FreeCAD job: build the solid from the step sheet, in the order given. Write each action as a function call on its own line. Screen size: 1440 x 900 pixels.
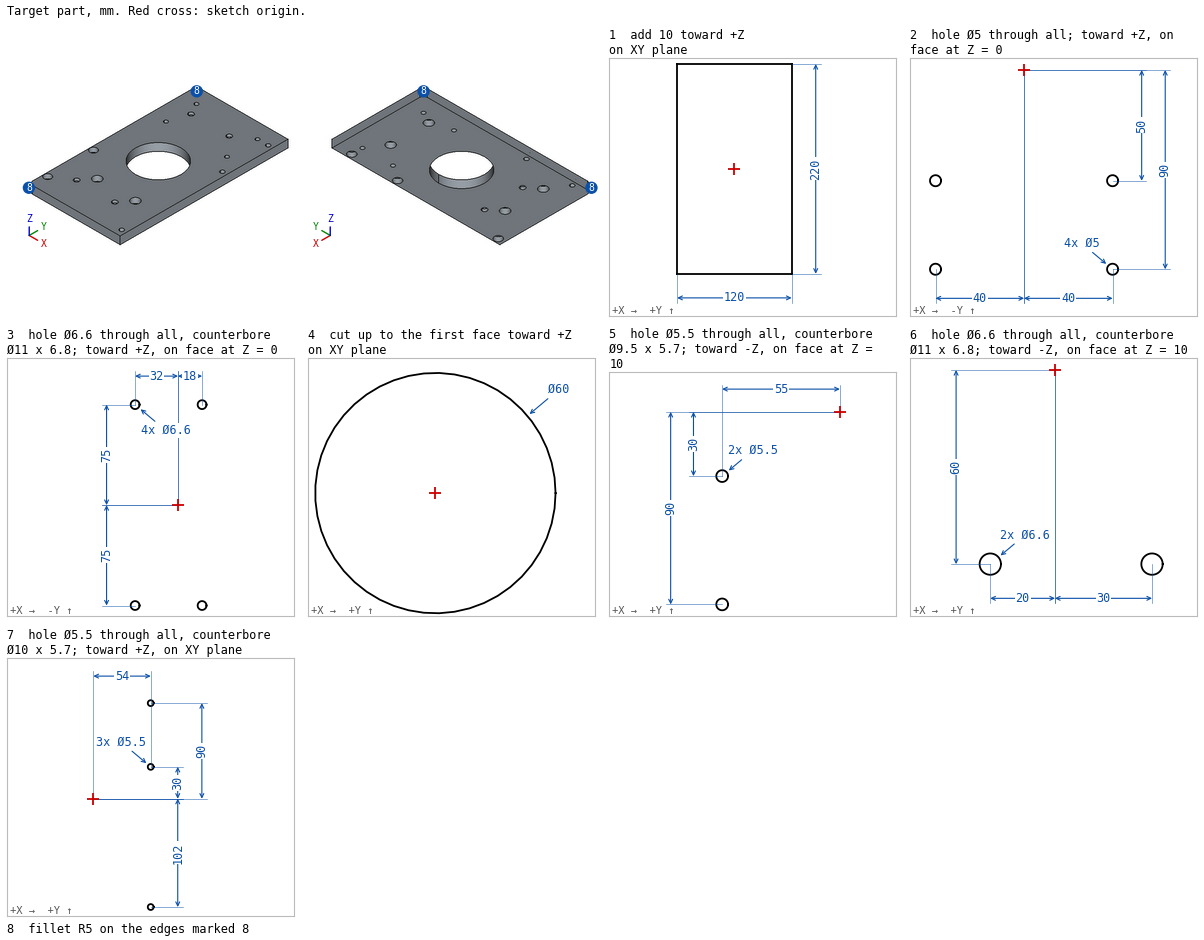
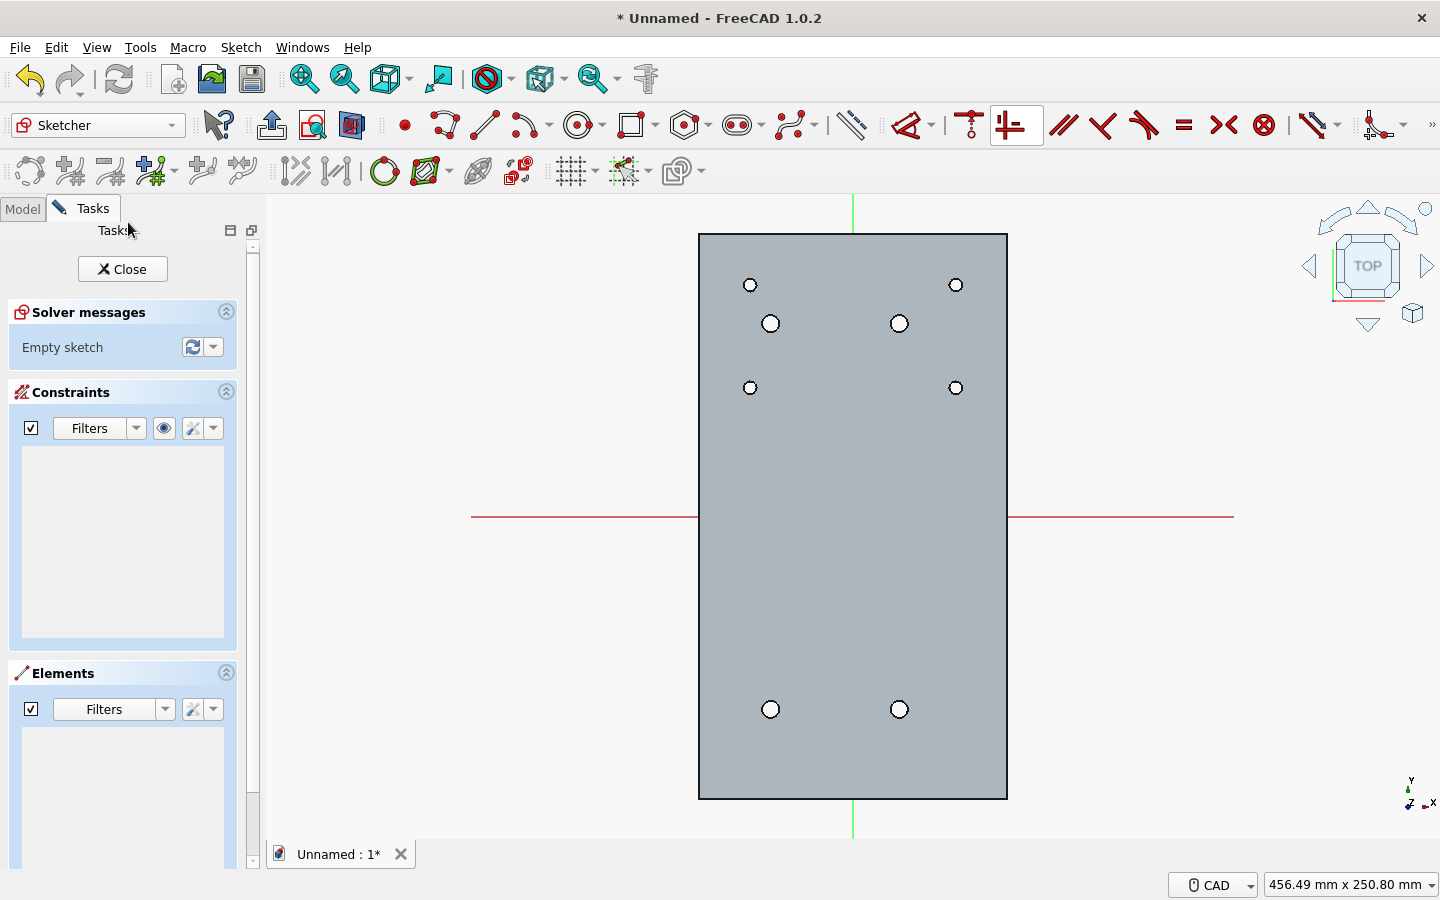
key(q)
key(s)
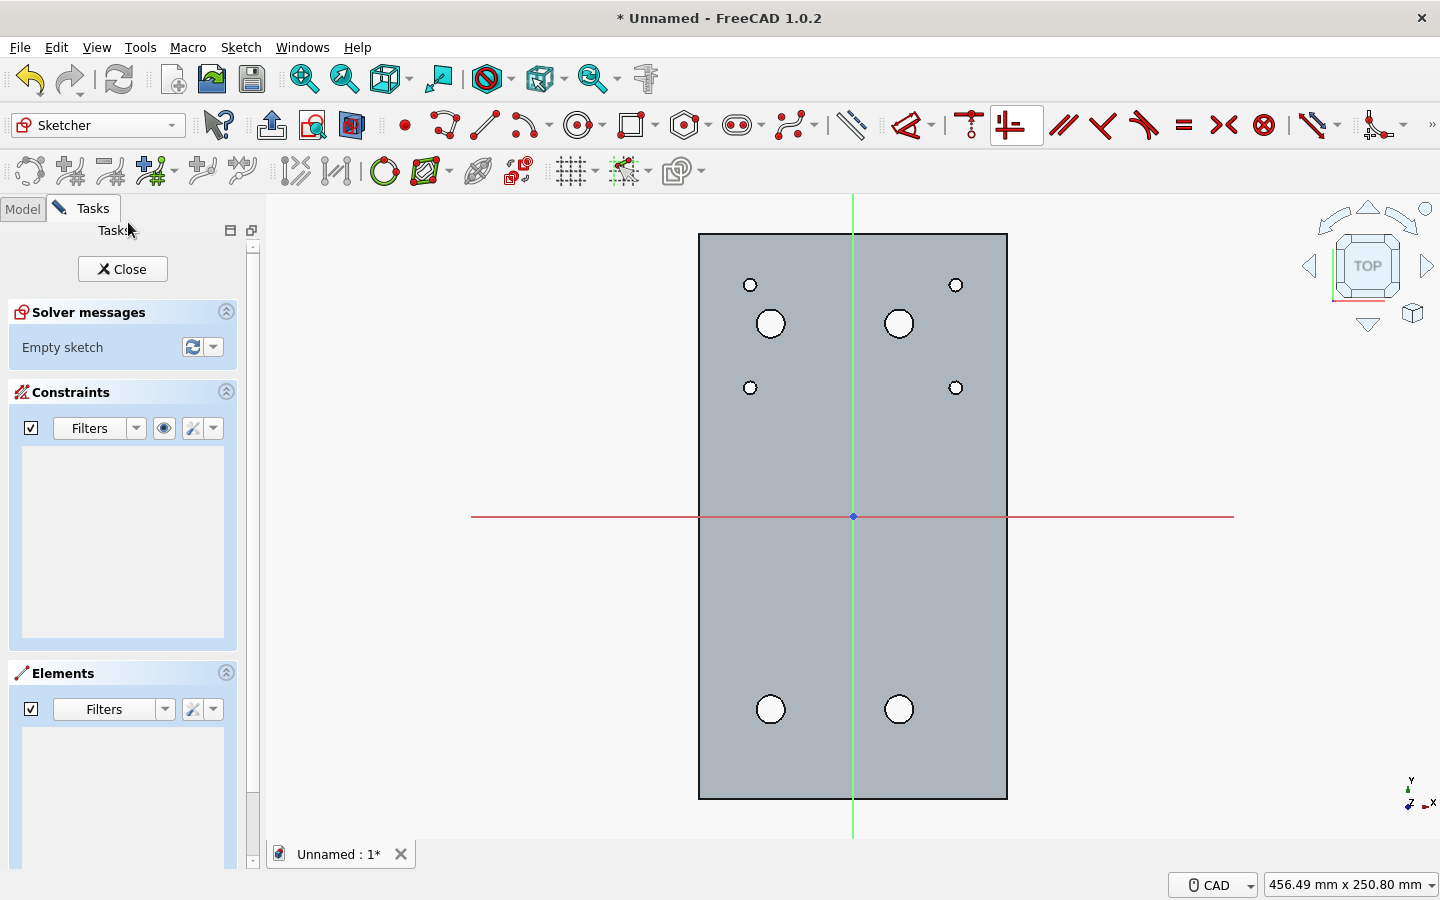
scroll(893, 516, up, 5)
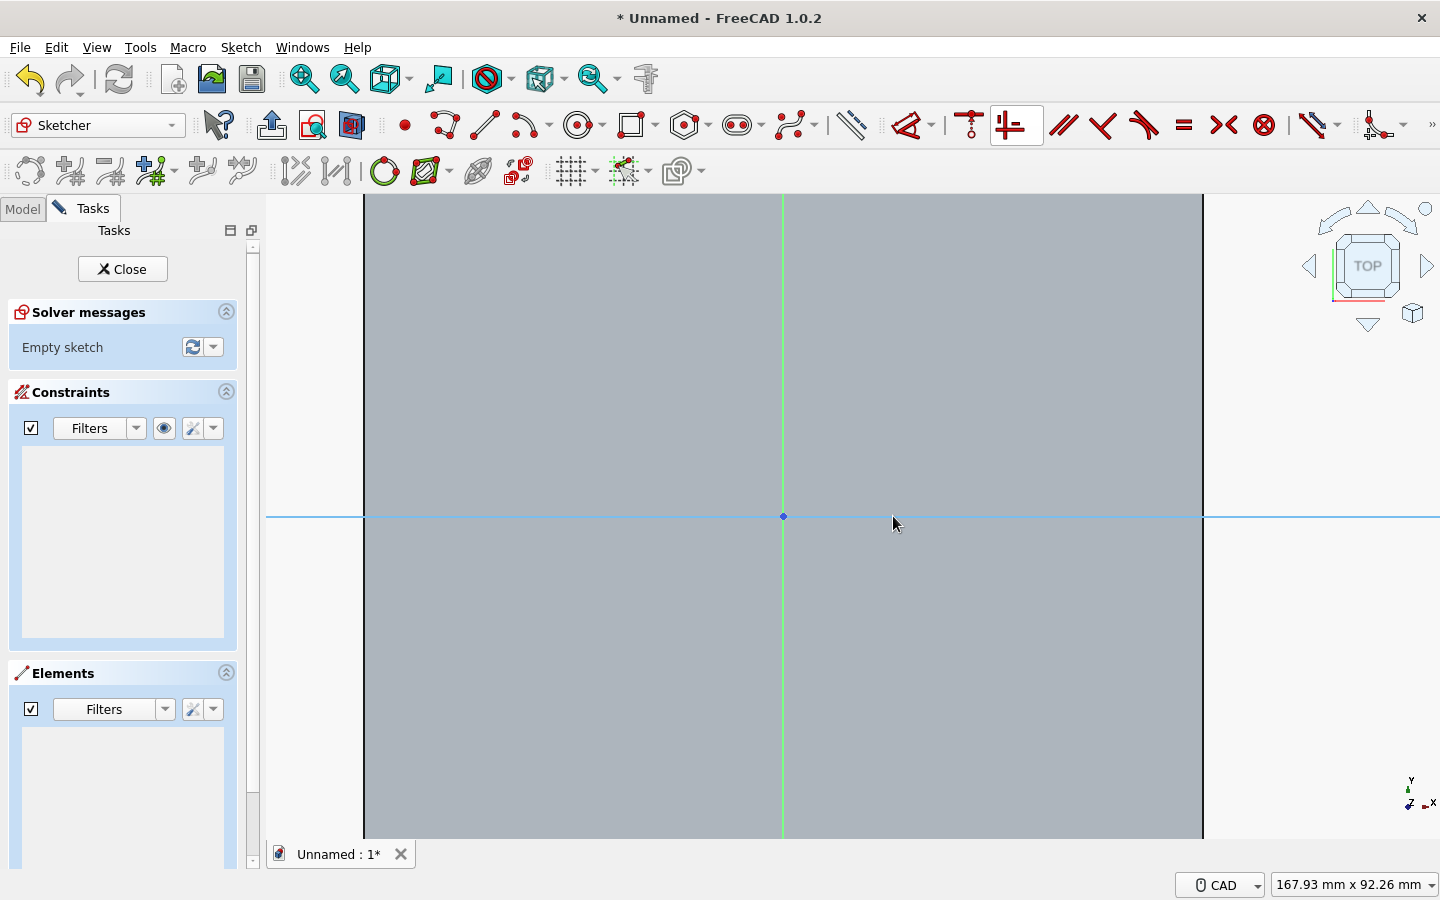
key(g)
key(c)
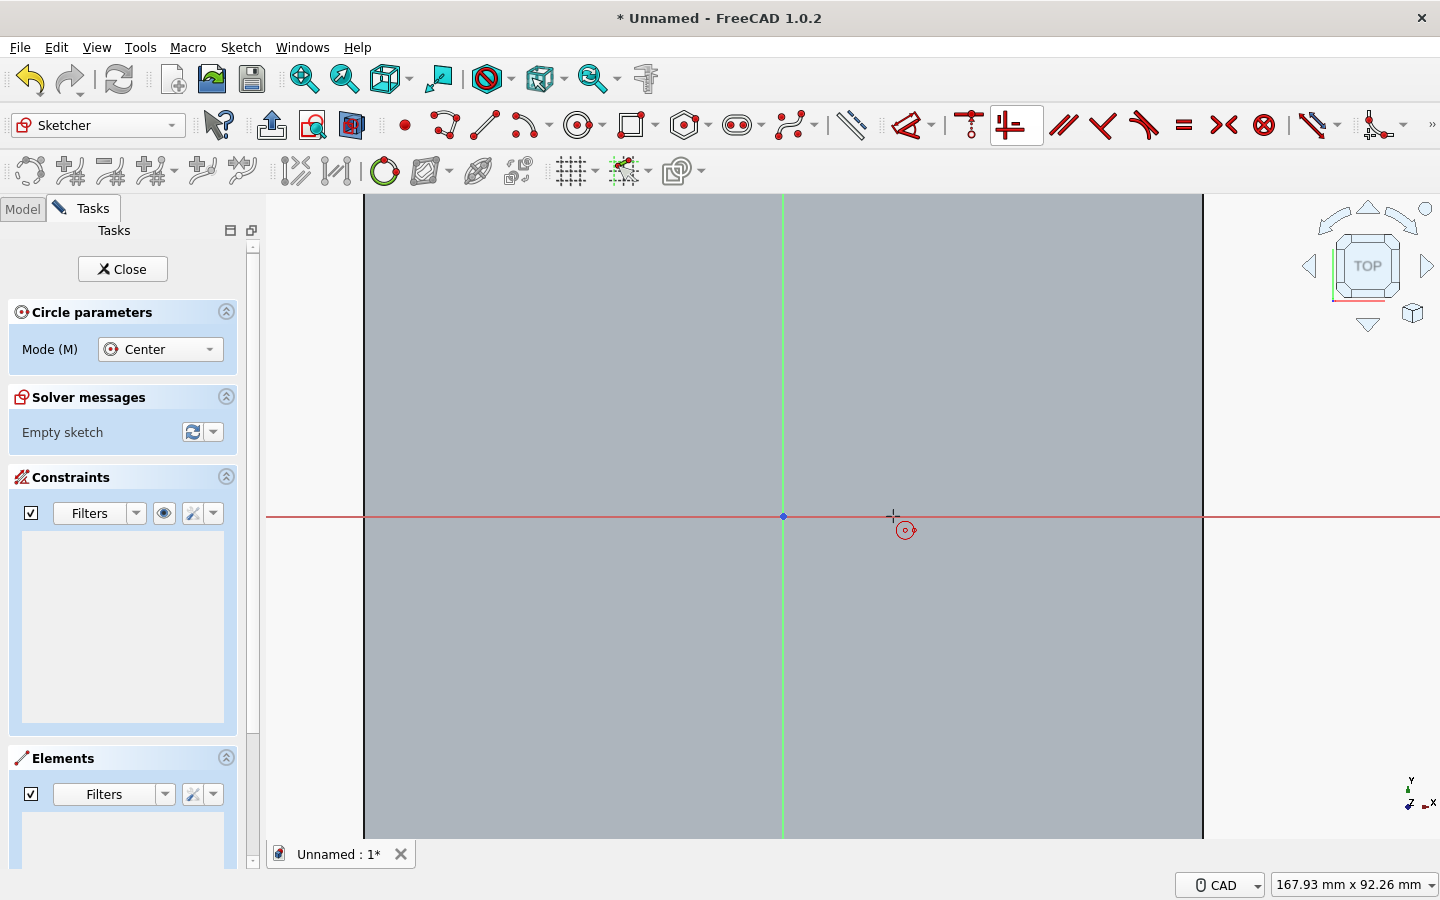
click(783, 516)
move(932, 368)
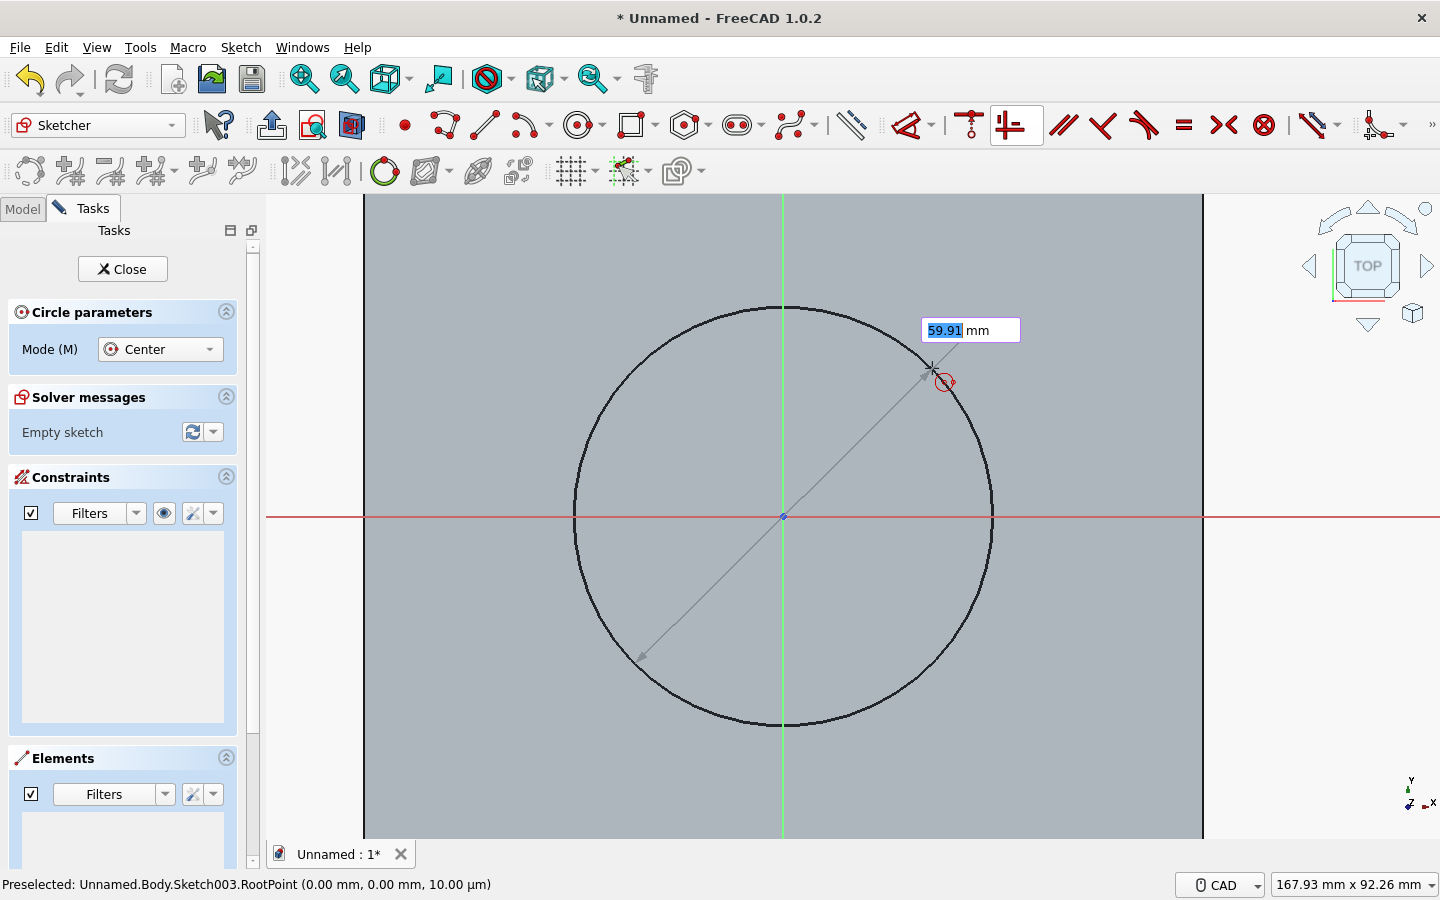
text(60)
key(Return)
key(Escape)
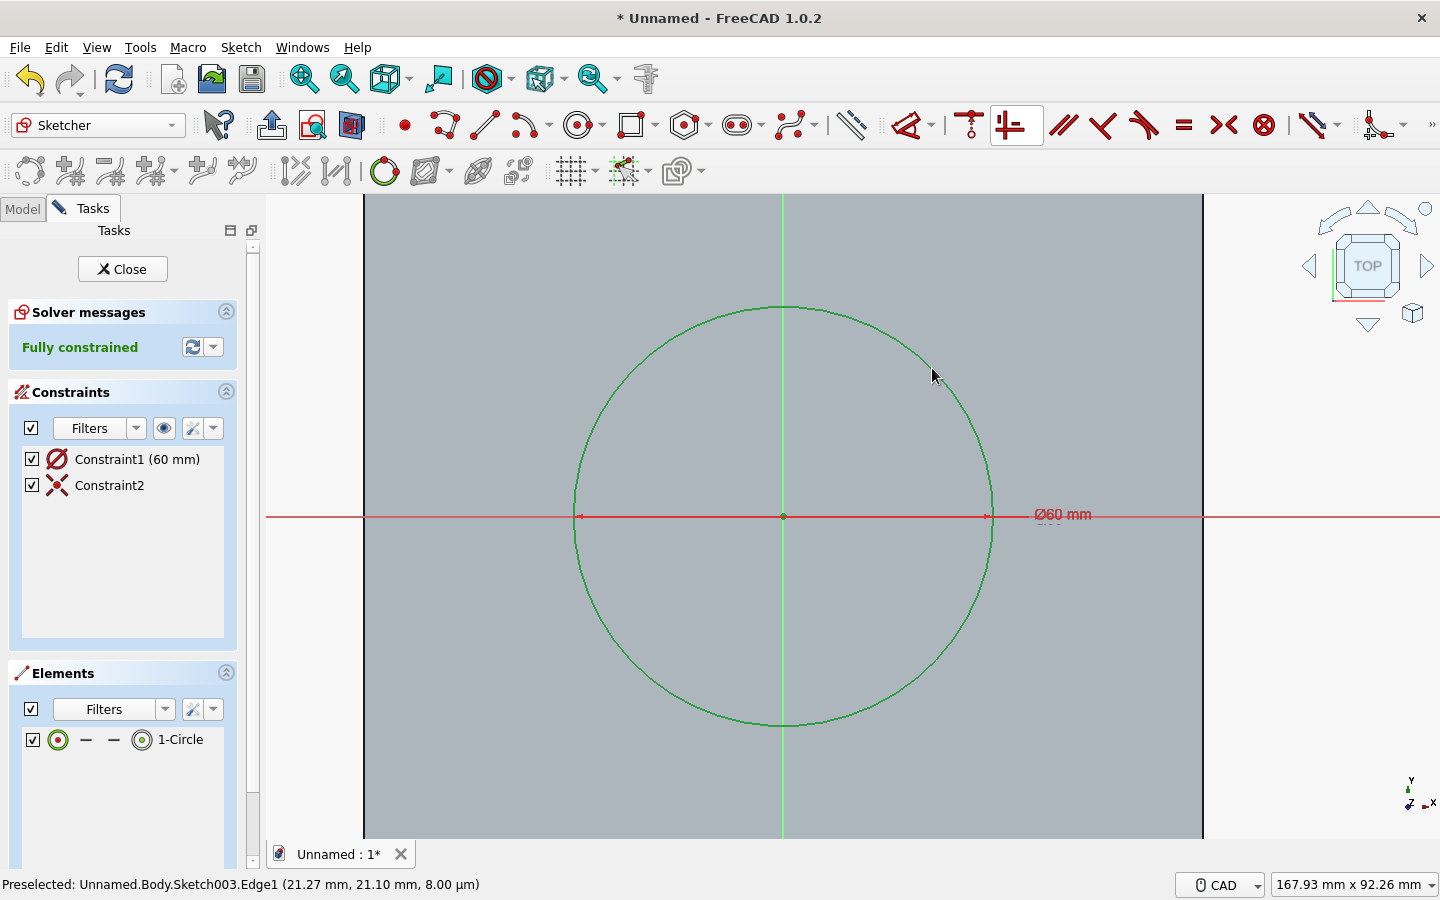
click(123, 269)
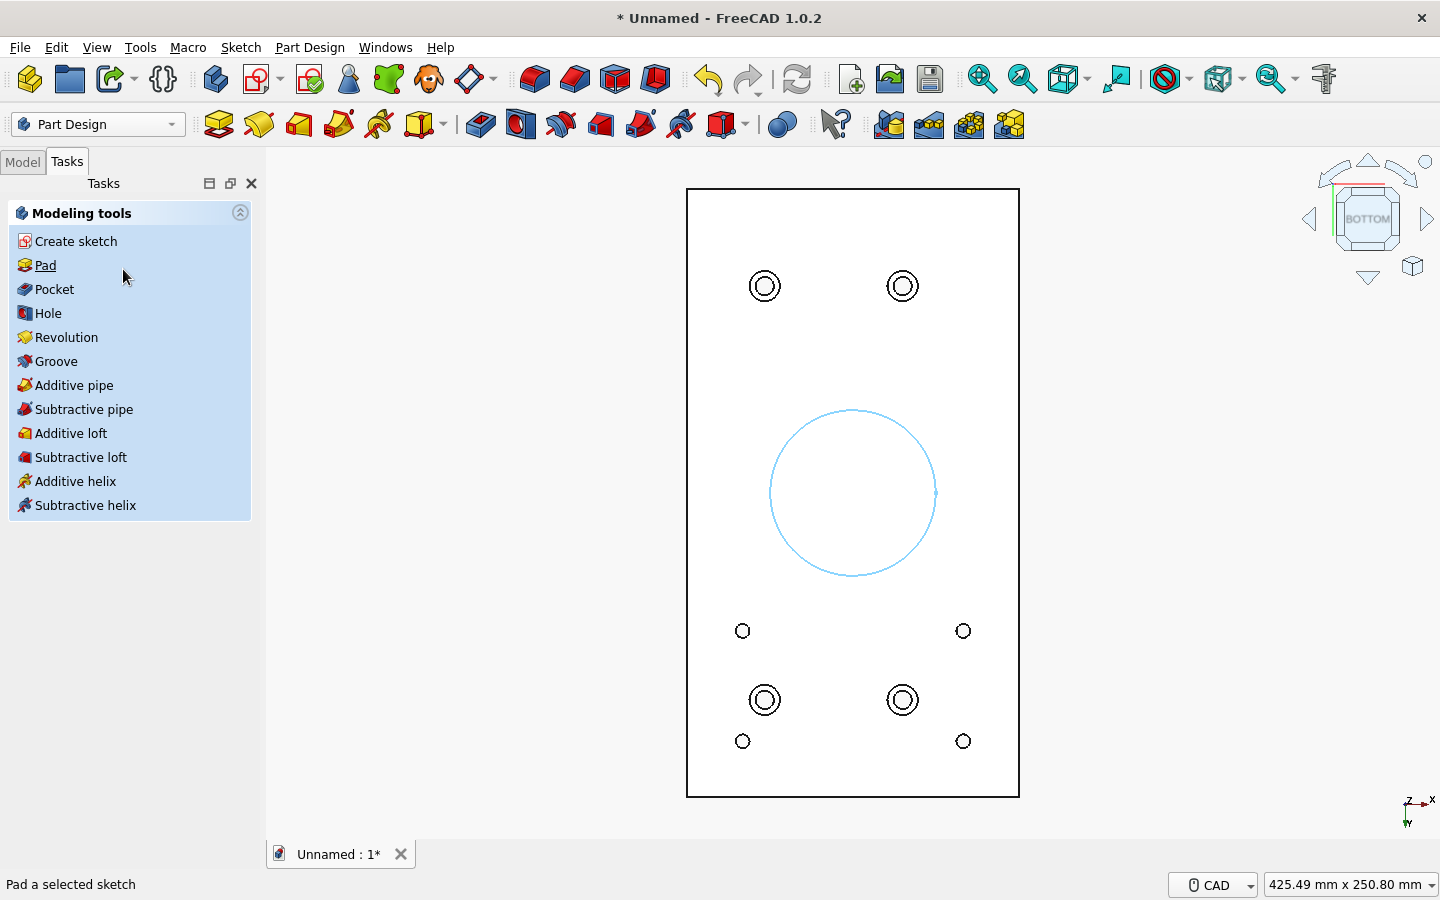
click(482, 124)